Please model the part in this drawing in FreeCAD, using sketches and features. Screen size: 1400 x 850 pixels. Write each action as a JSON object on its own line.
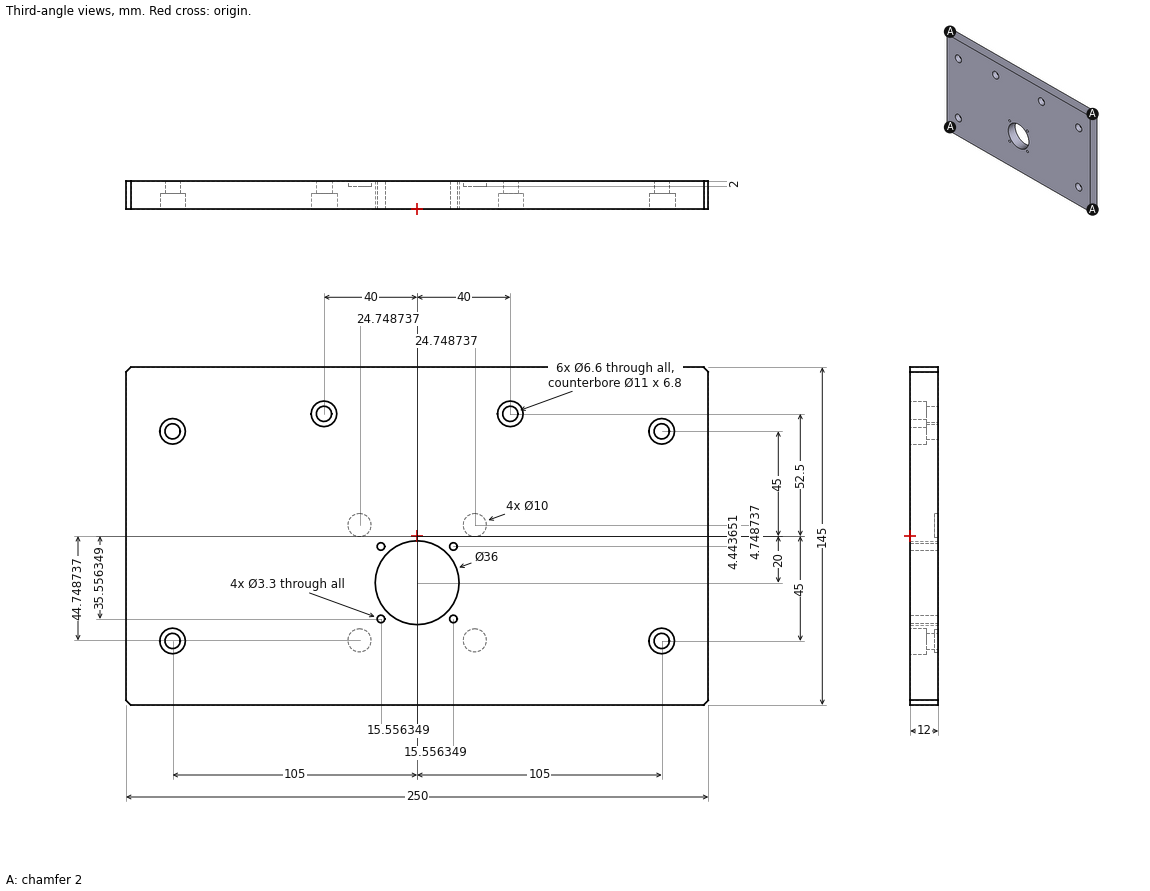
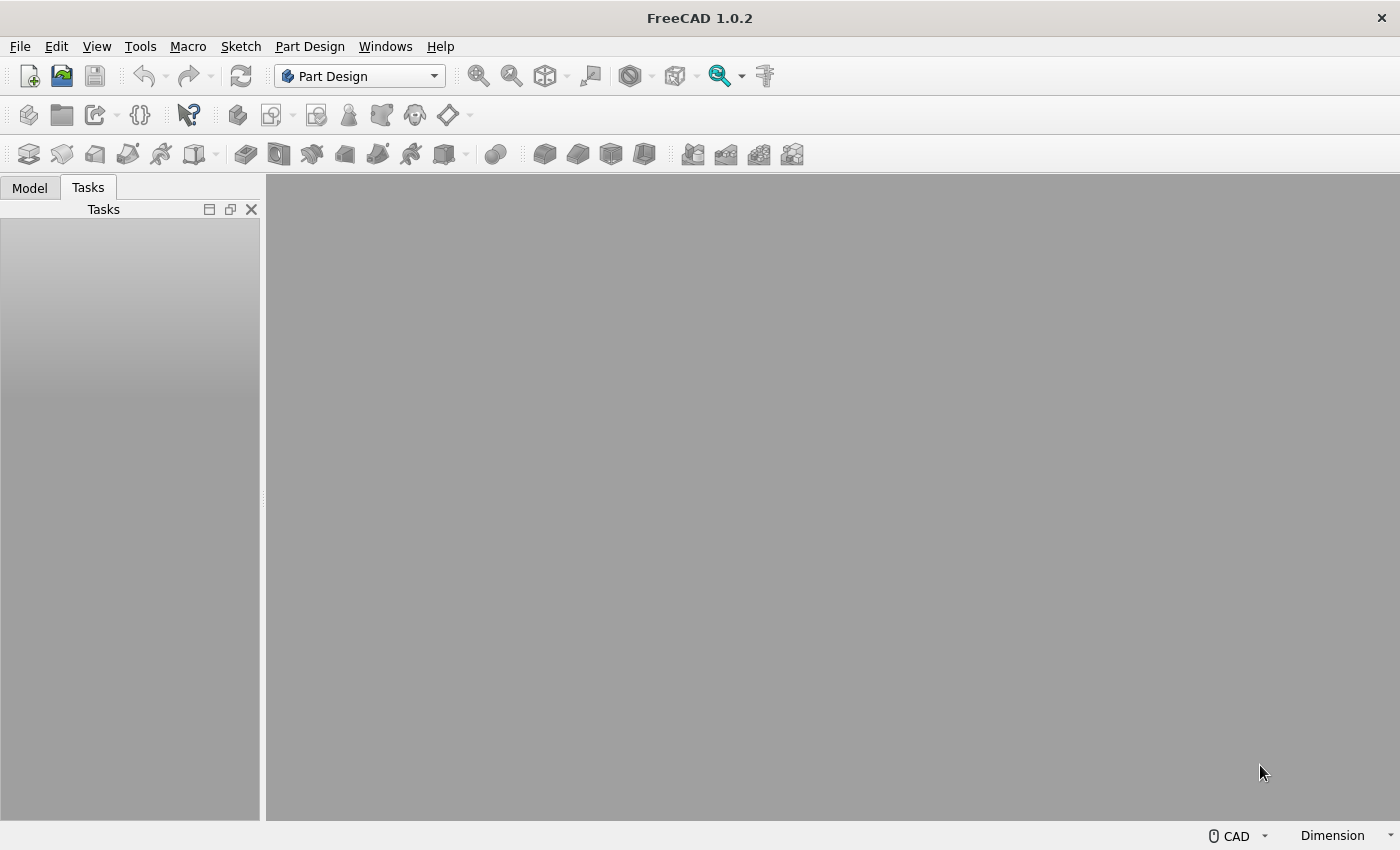
{"action": "left_click", "coordinate": [29, 76]}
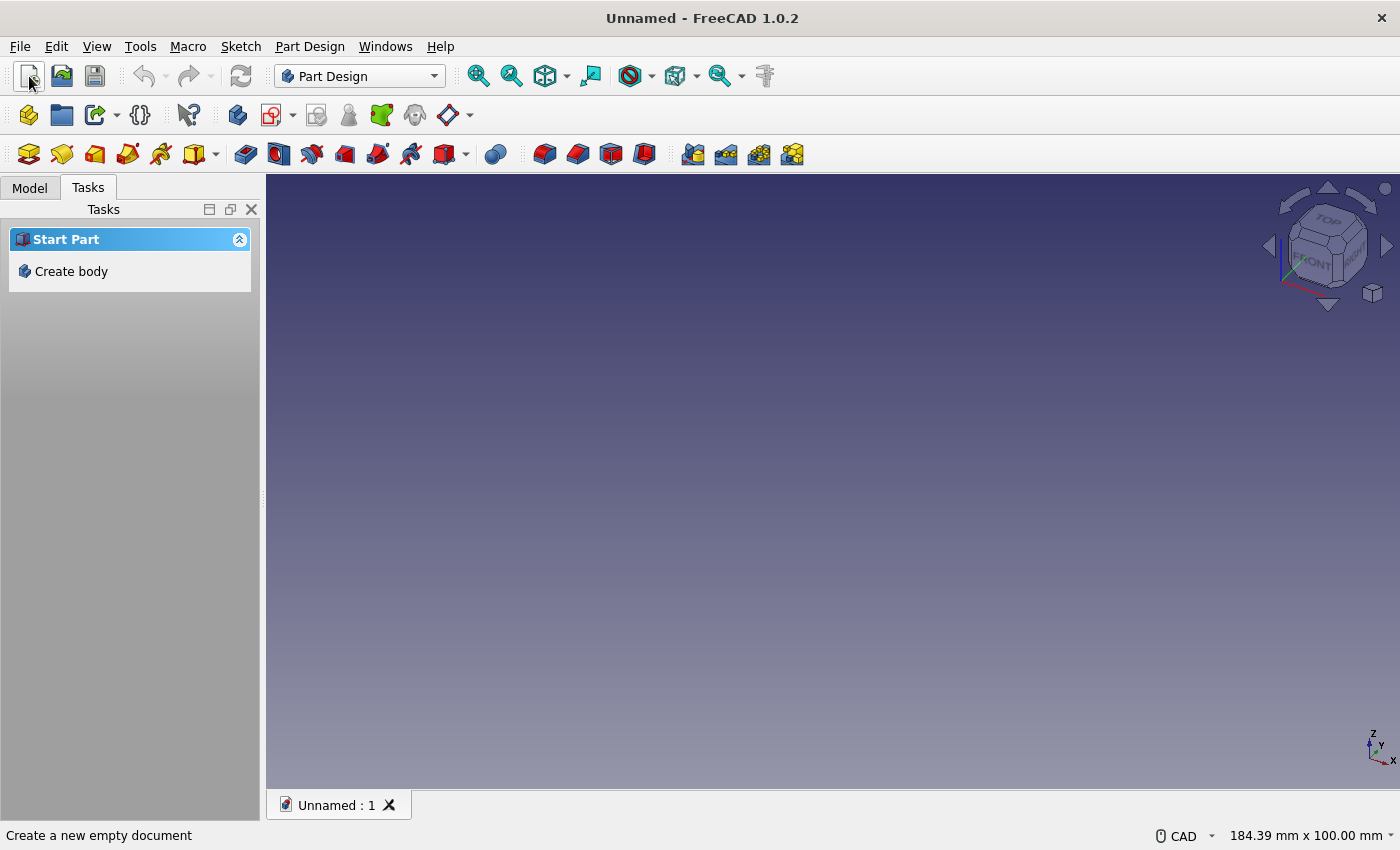
{"action": "left_click", "coordinate": [270, 116]}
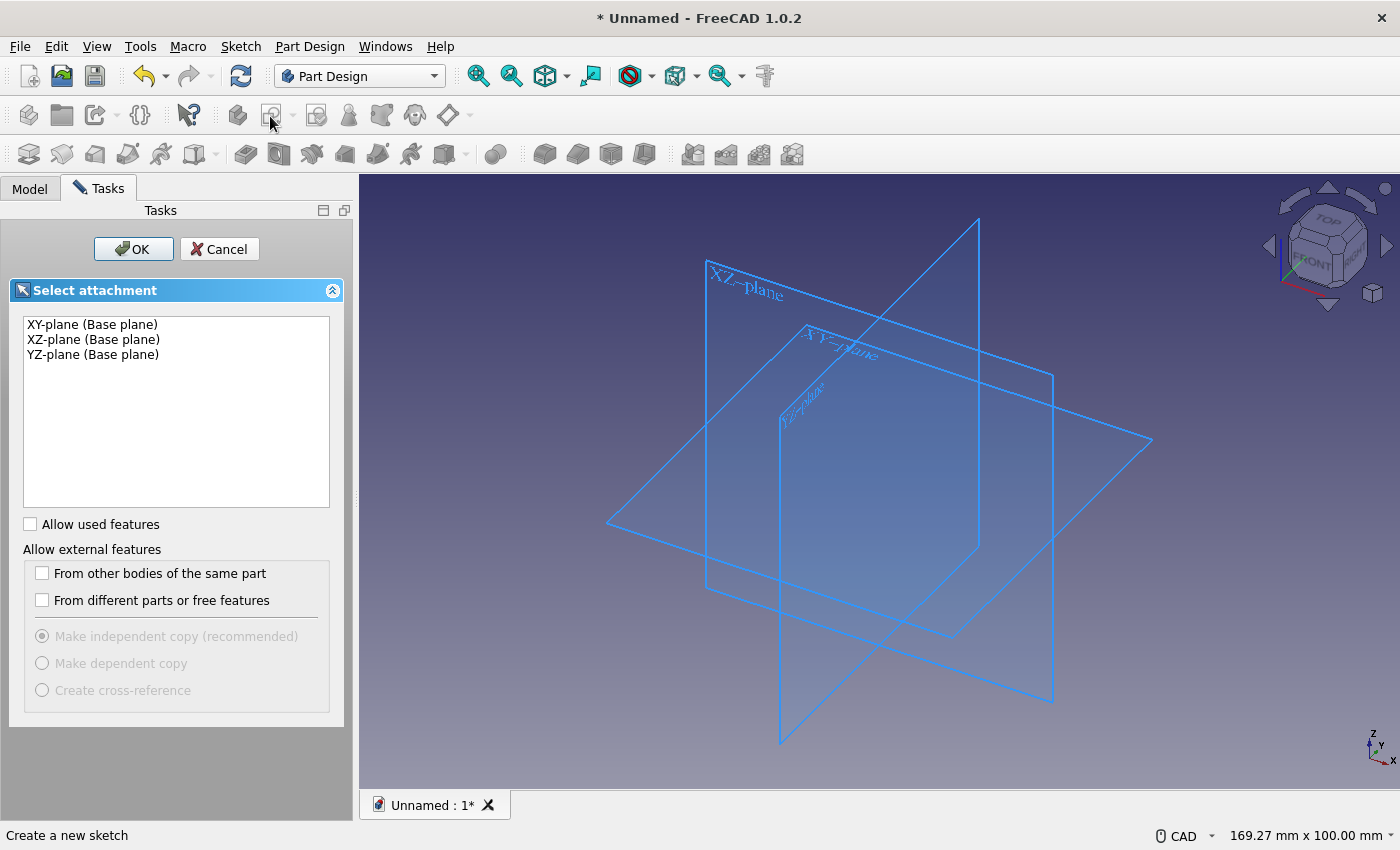
{"action": "left_click", "coordinate": [84, 340]}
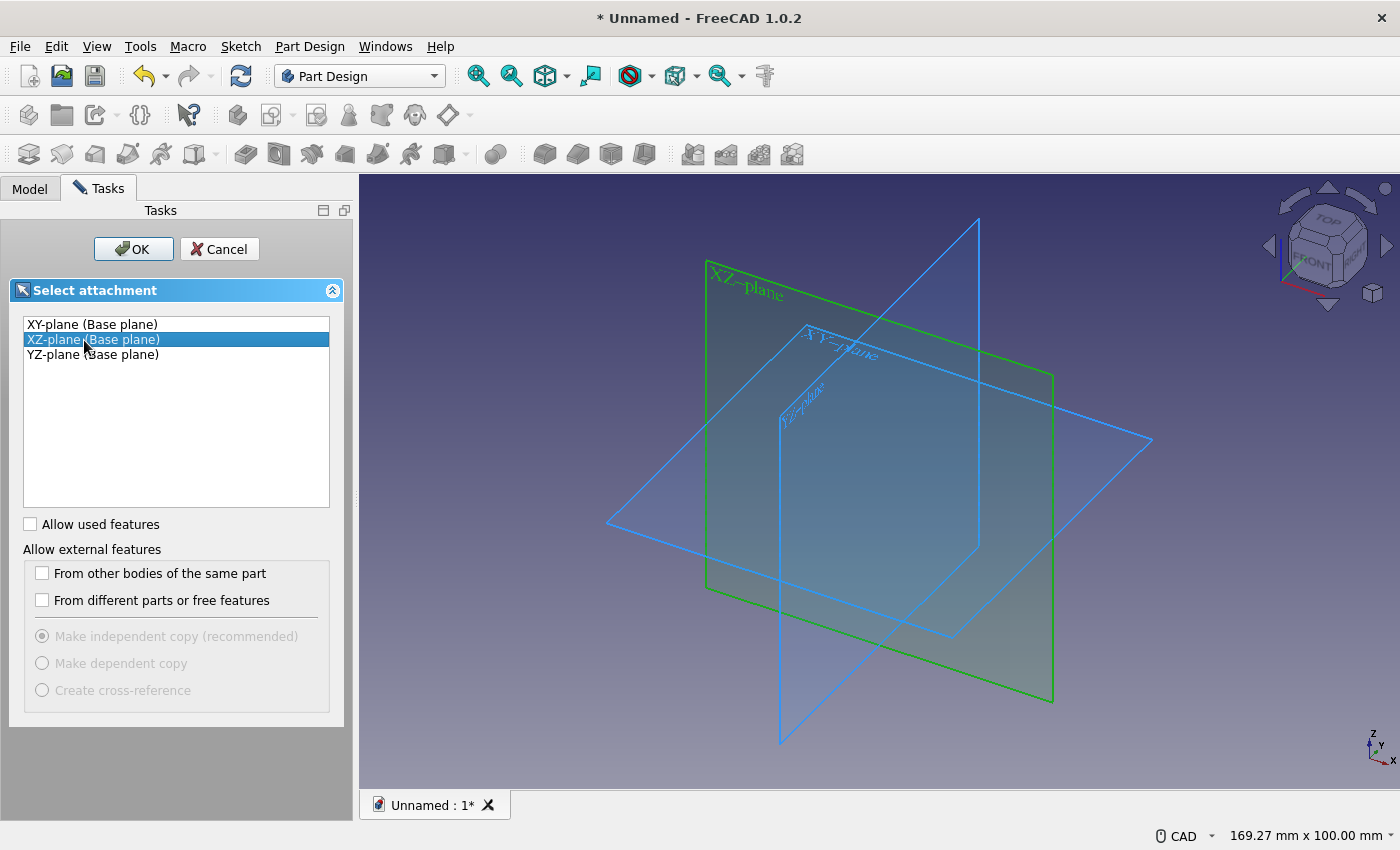
{"action": "left_click", "coordinate": [134, 249]}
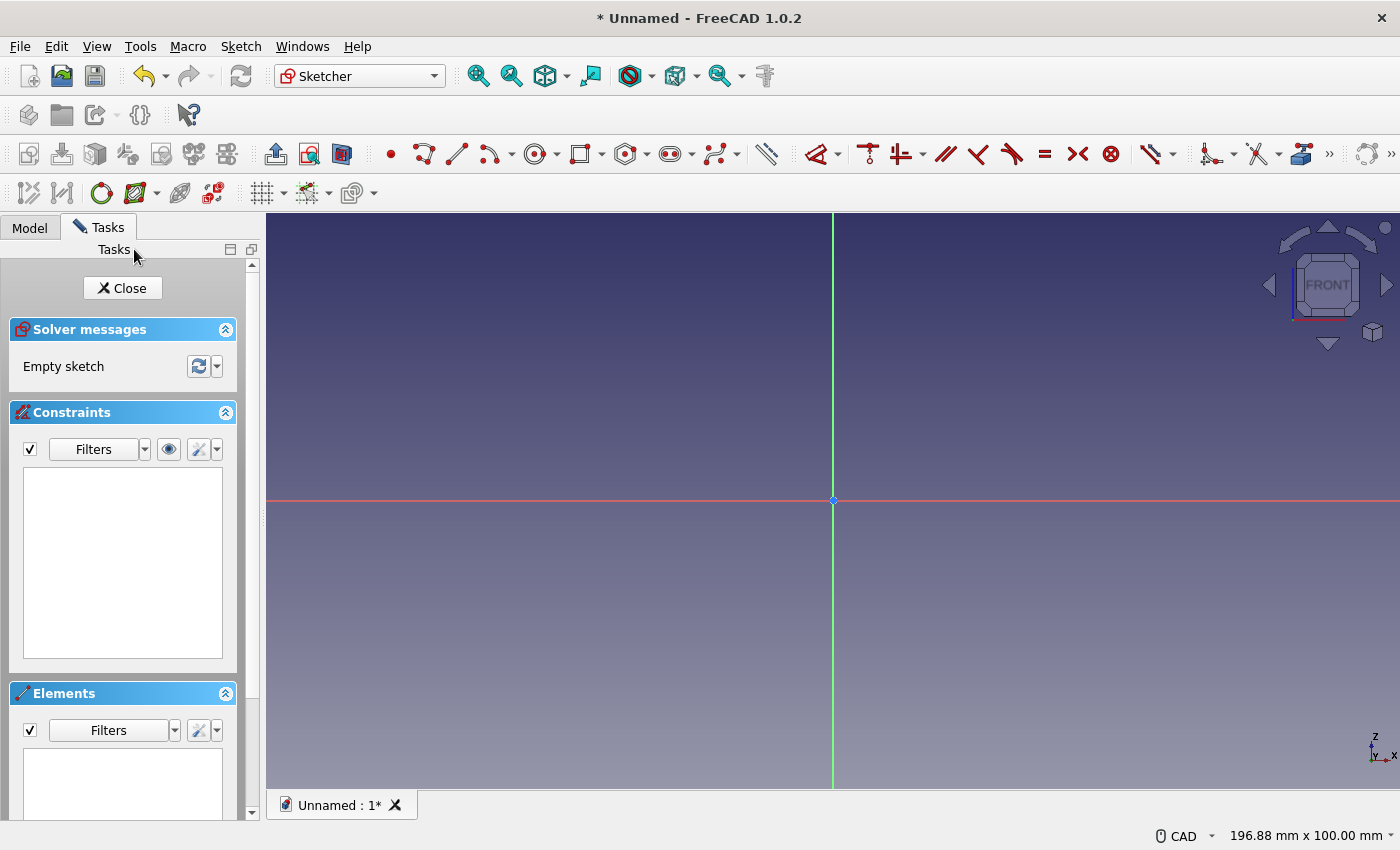
{"action": "scroll", "coordinate": [709, 501], "scroll_direction": "down", "scroll_amount": 4}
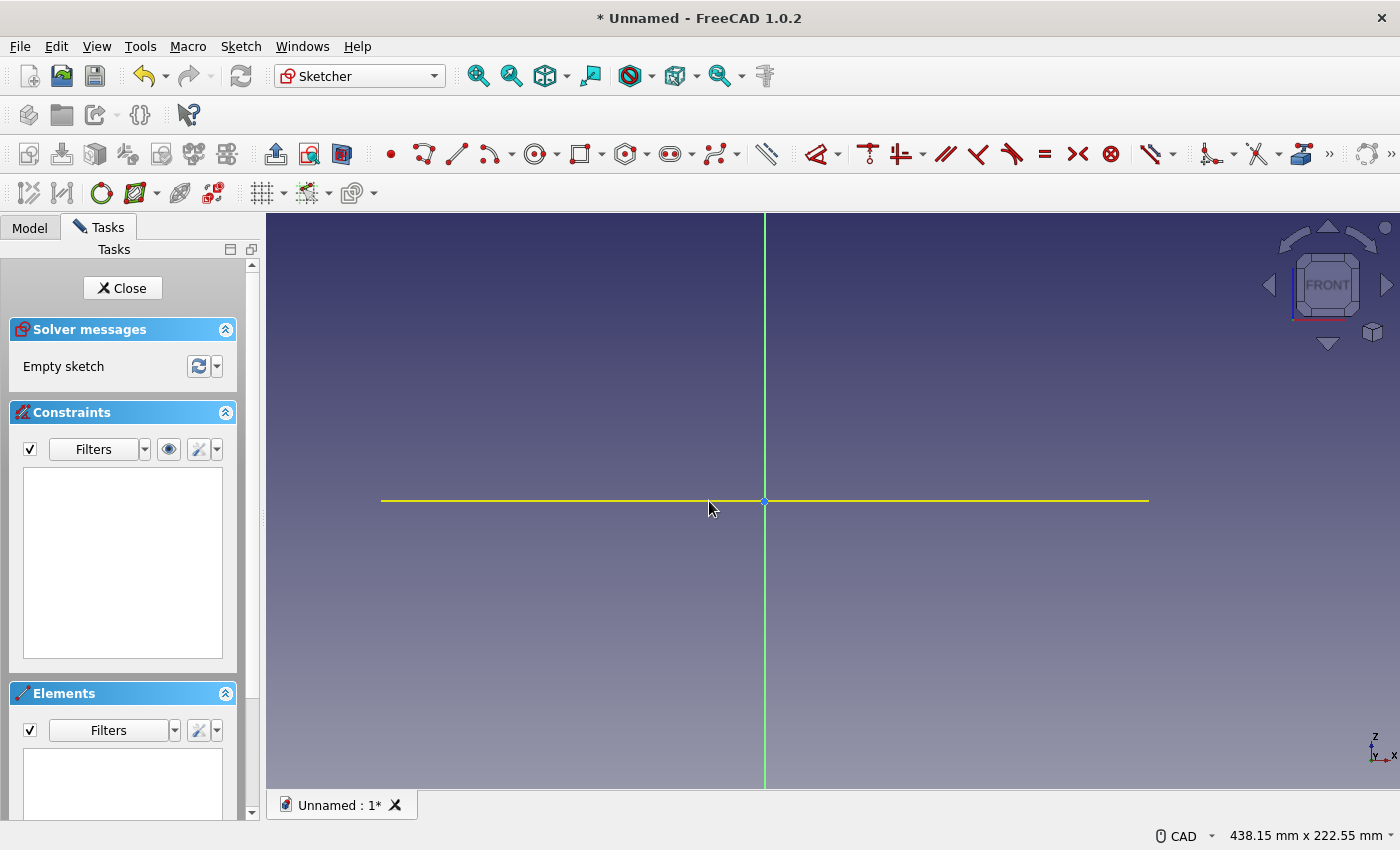
{"action": "left_click", "coordinate": [602, 154]}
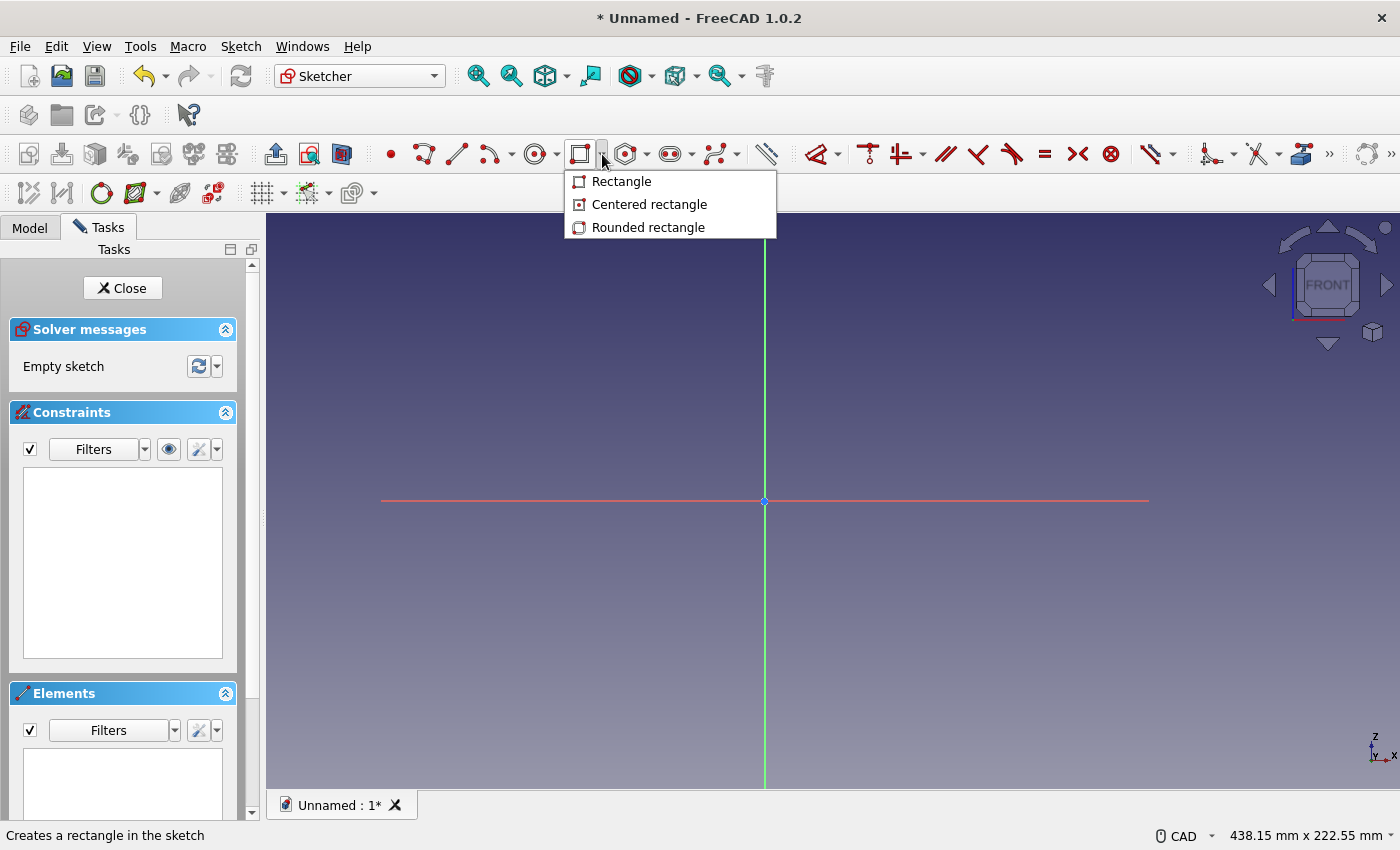
{"action": "left_click", "coordinate": [670, 204]}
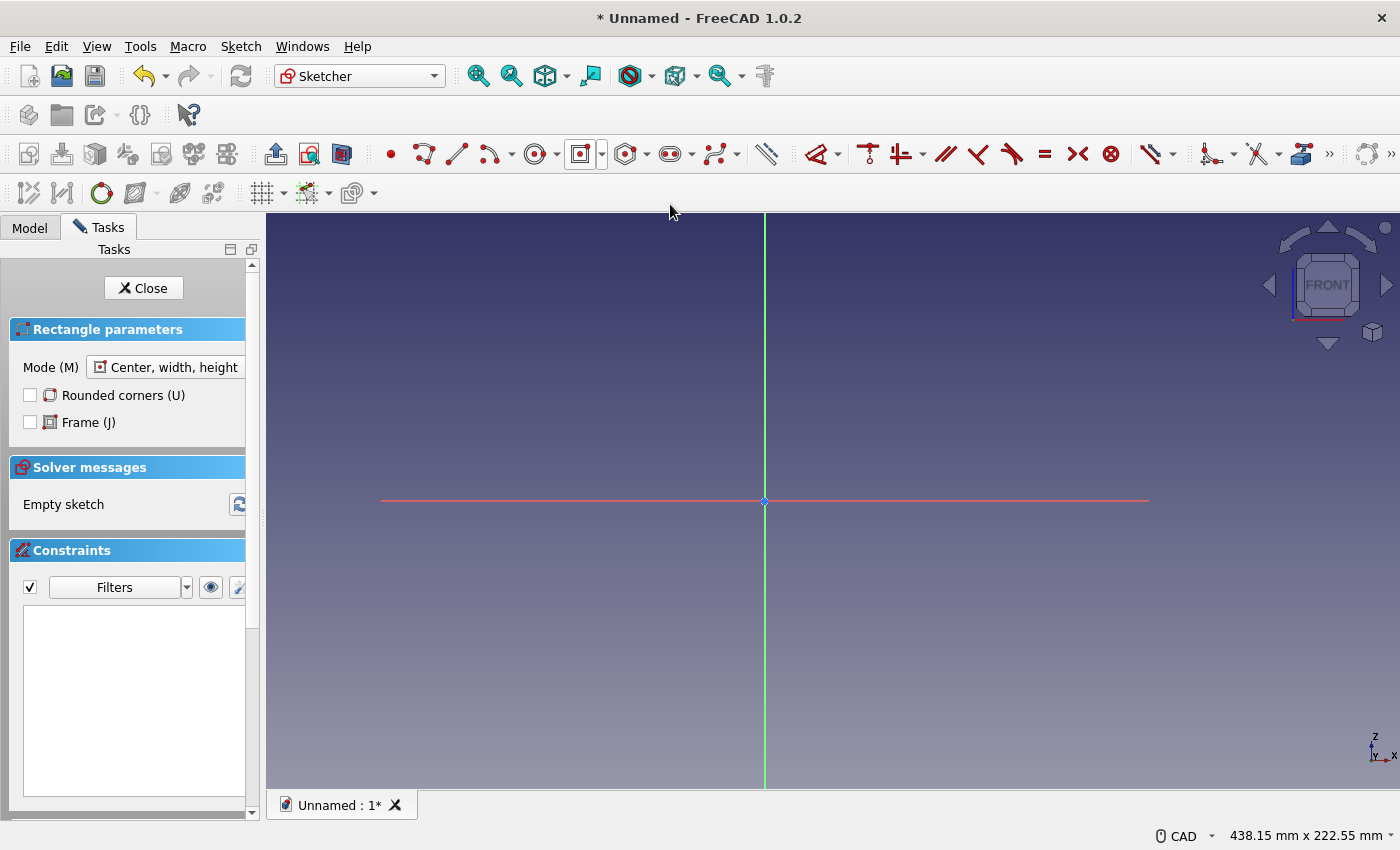
{"action": "left_click", "coordinate": [765, 501]}
{"action": "mouse_move", "coordinate": [1088, 314]}